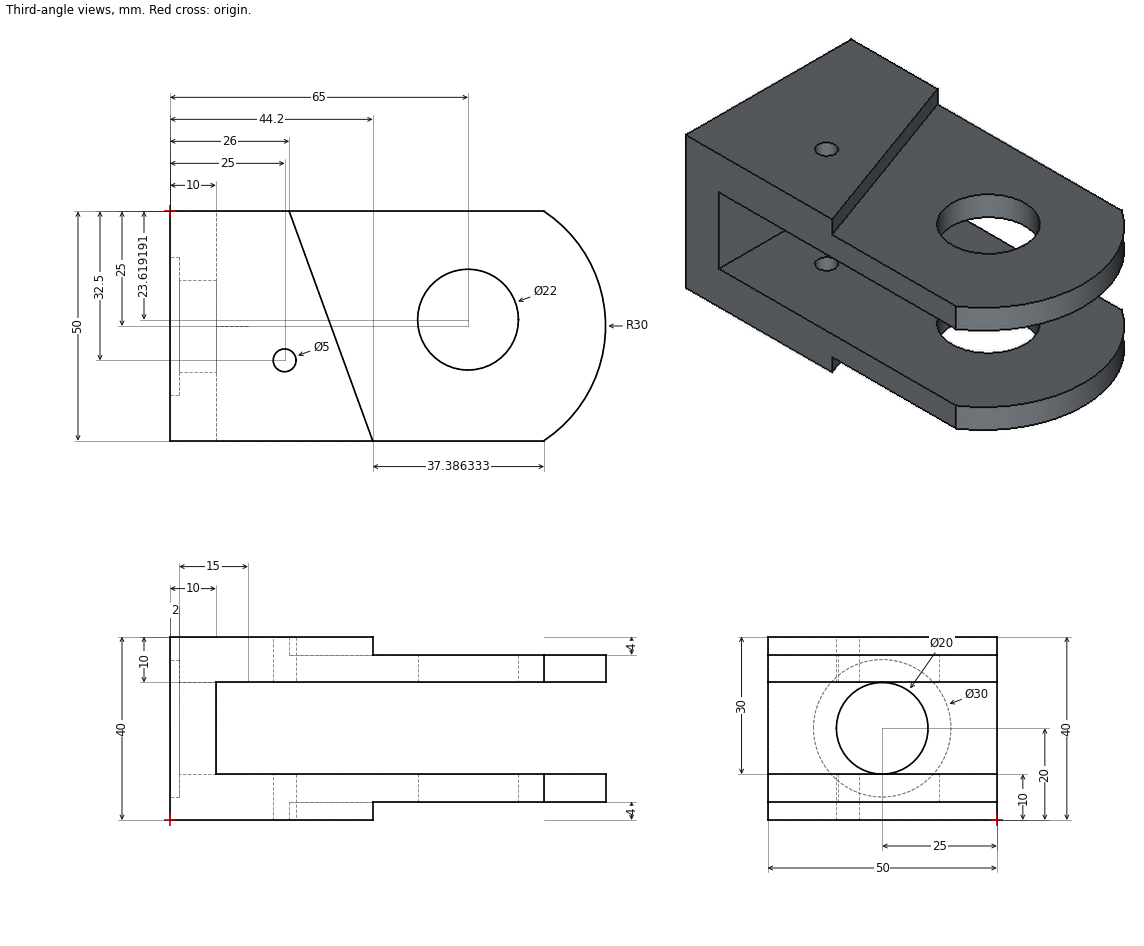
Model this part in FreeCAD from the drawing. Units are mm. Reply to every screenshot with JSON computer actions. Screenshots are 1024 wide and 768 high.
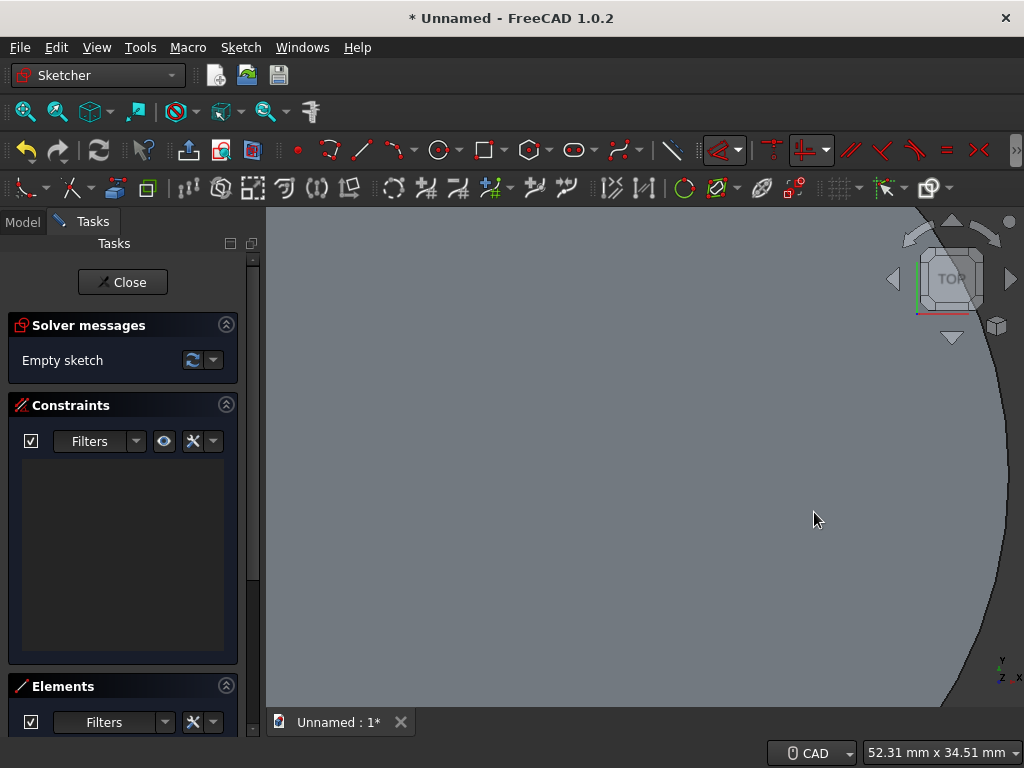
{"action": "left_click", "coordinate": [440, 150]}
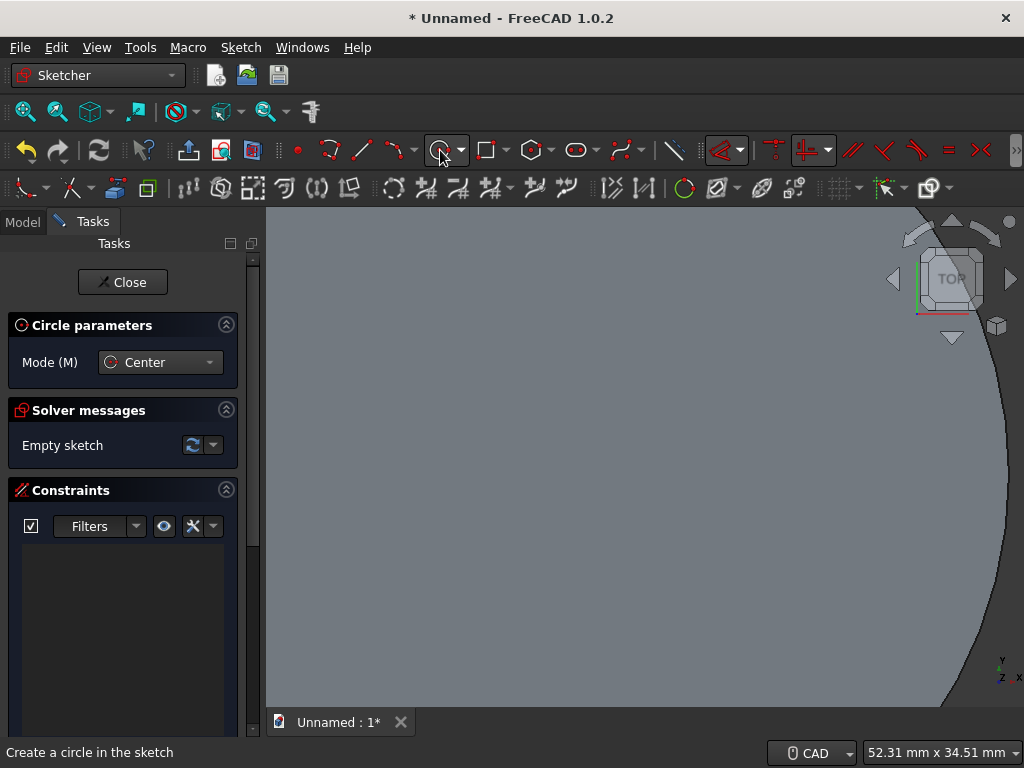
{"action": "left_click", "coordinate": [574, 454]}
{"action": "mouse_move", "coordinate": [687, 342]}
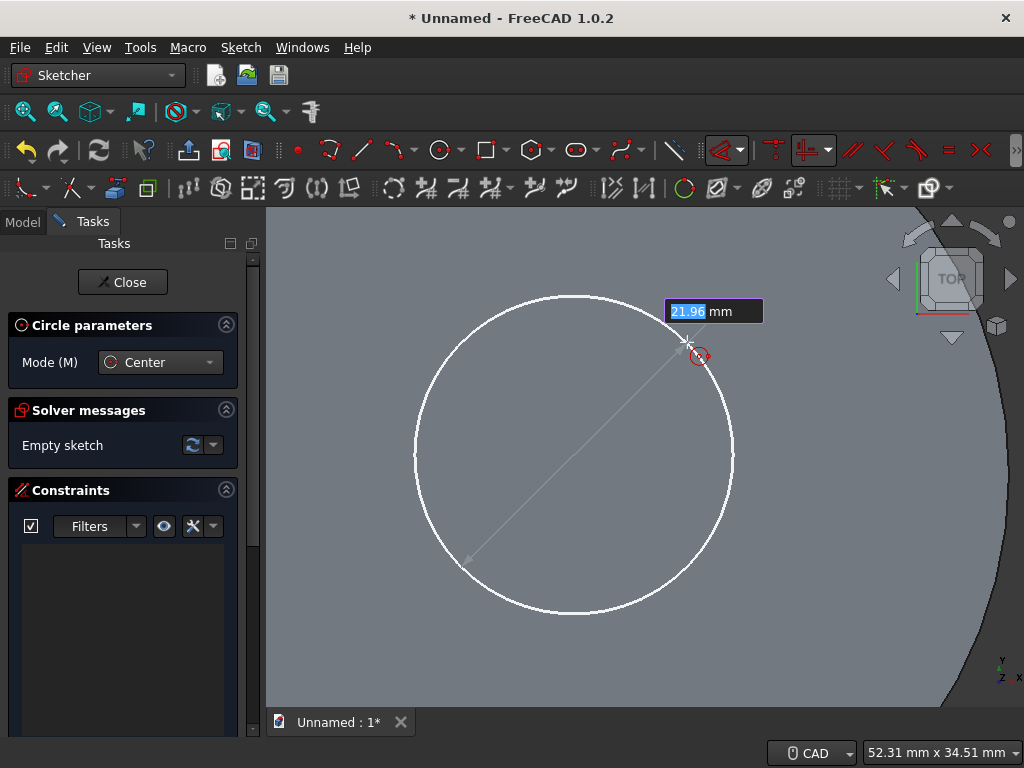
{"action": "type", "text": "22"}
{"action": "key", "text": "Return"}
{"action": "key", "text": "Escape"}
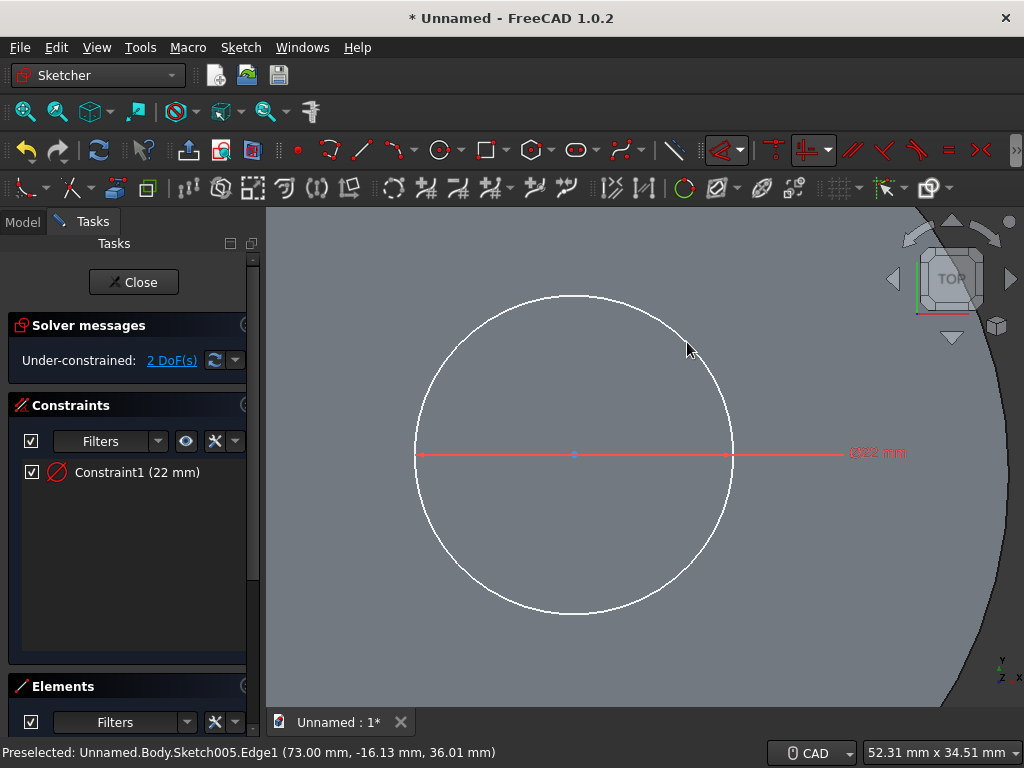
{"action": "left_click", "coordinate": [574, 455]}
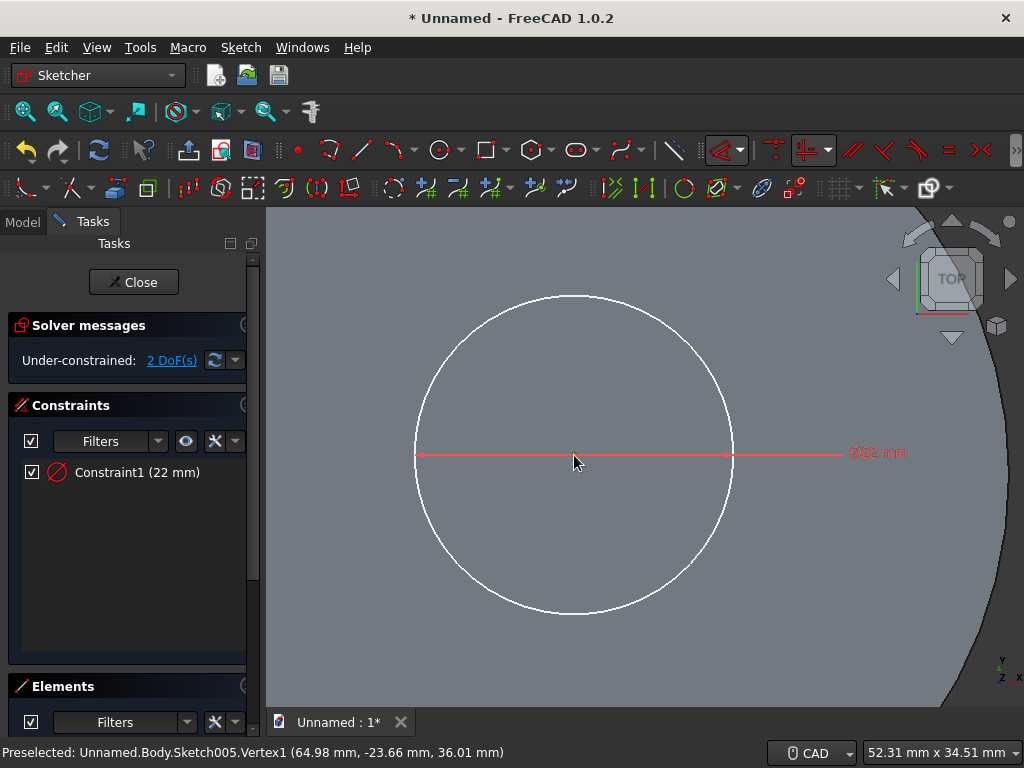
{"action": "key", "text": "l"}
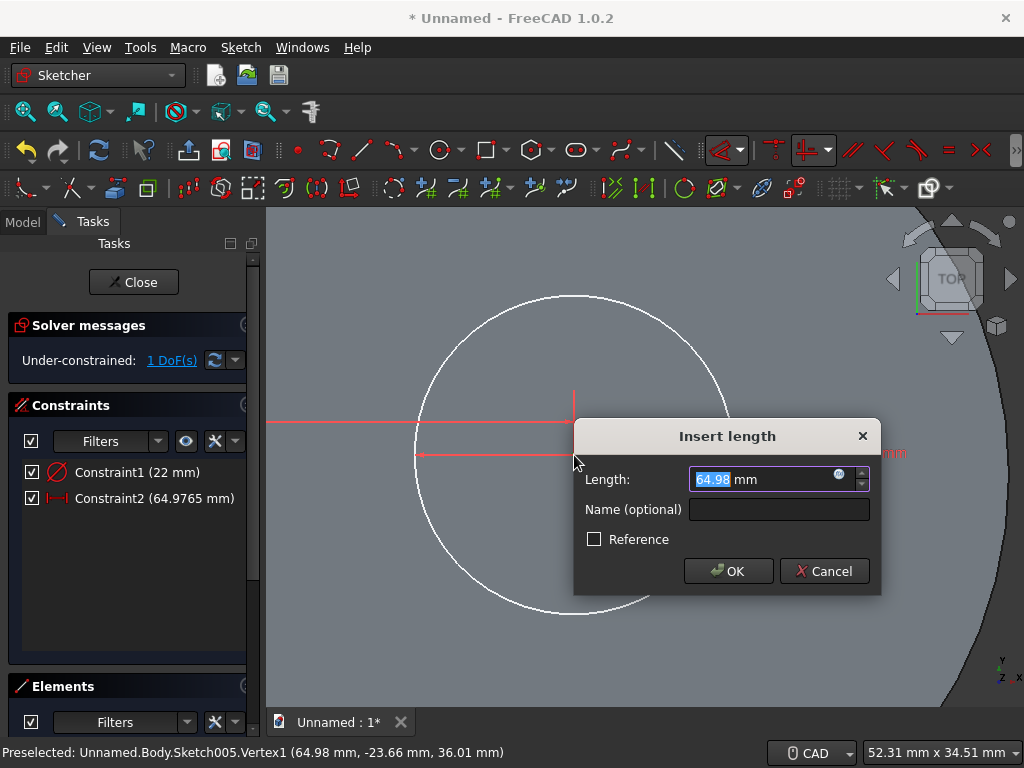
{"action": "type", "text": "65"}
{"action": "key", "text": "Return"}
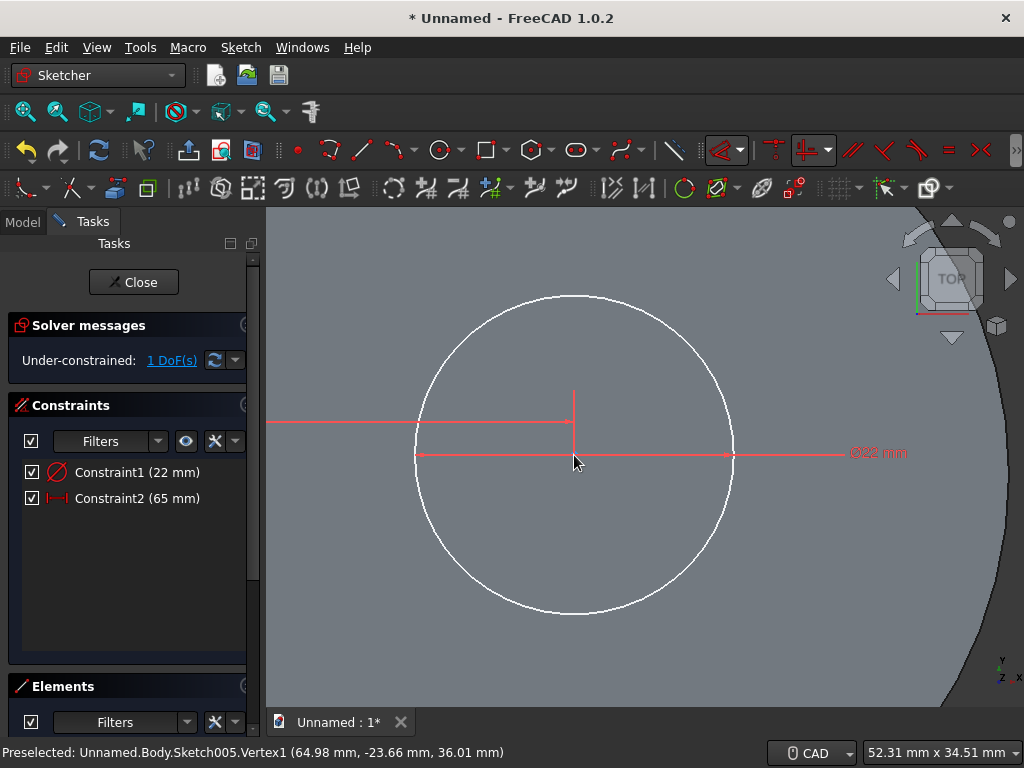
{"action": "left_click", "coordinate": [574, 455]}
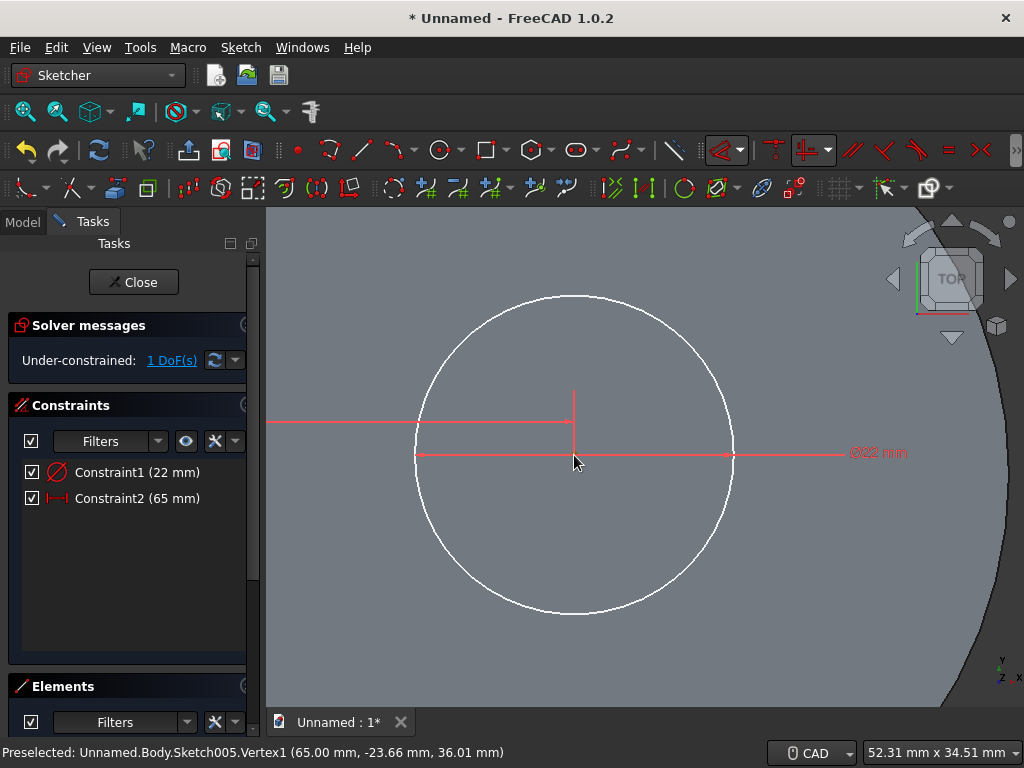
{"action": "key", "text": "i"}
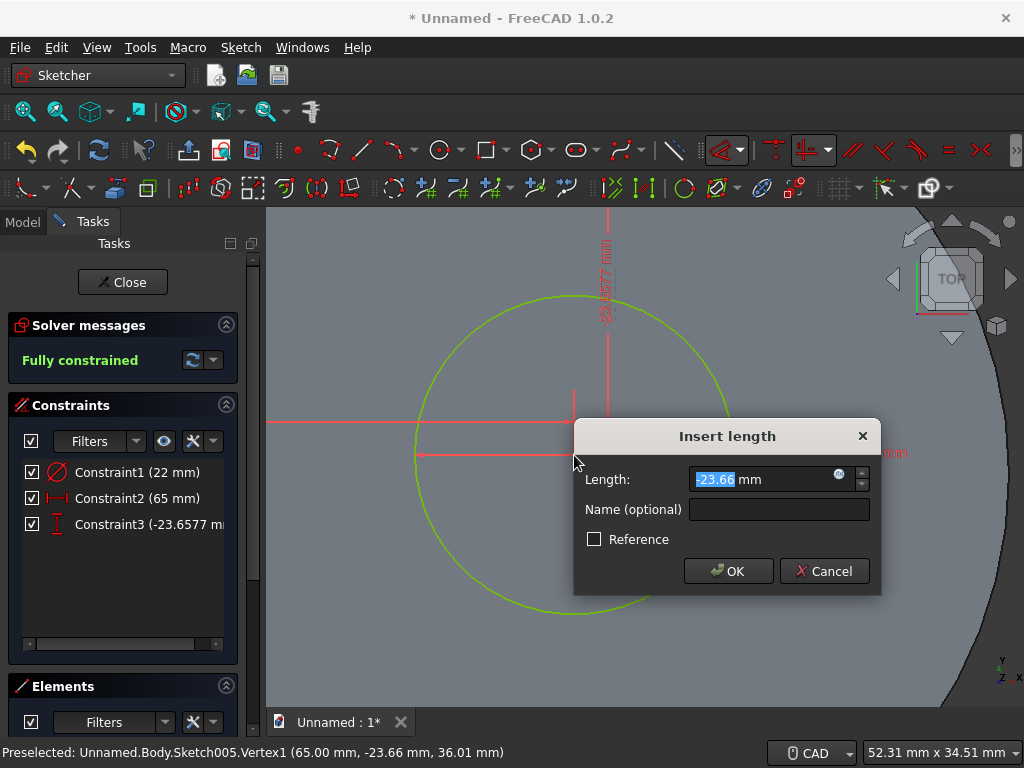
{"action": "type", "text": "-23.619191"}
{"action": "key", "text": "Return"}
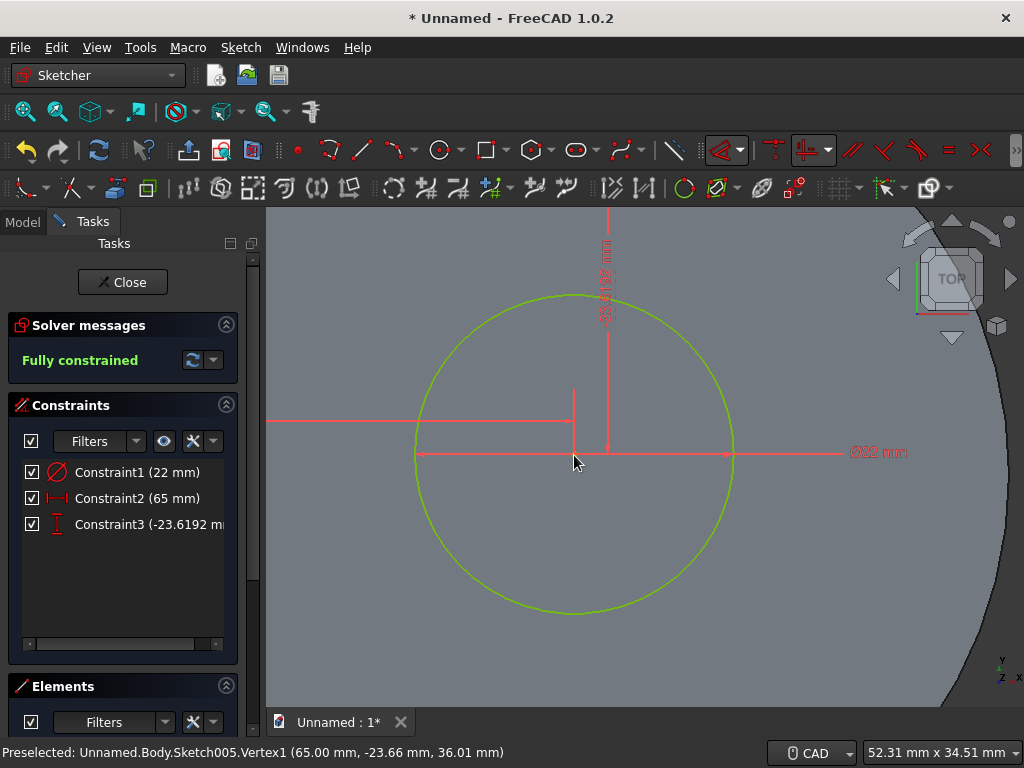
{"action": "left_click", "coordinate": [123, 282]}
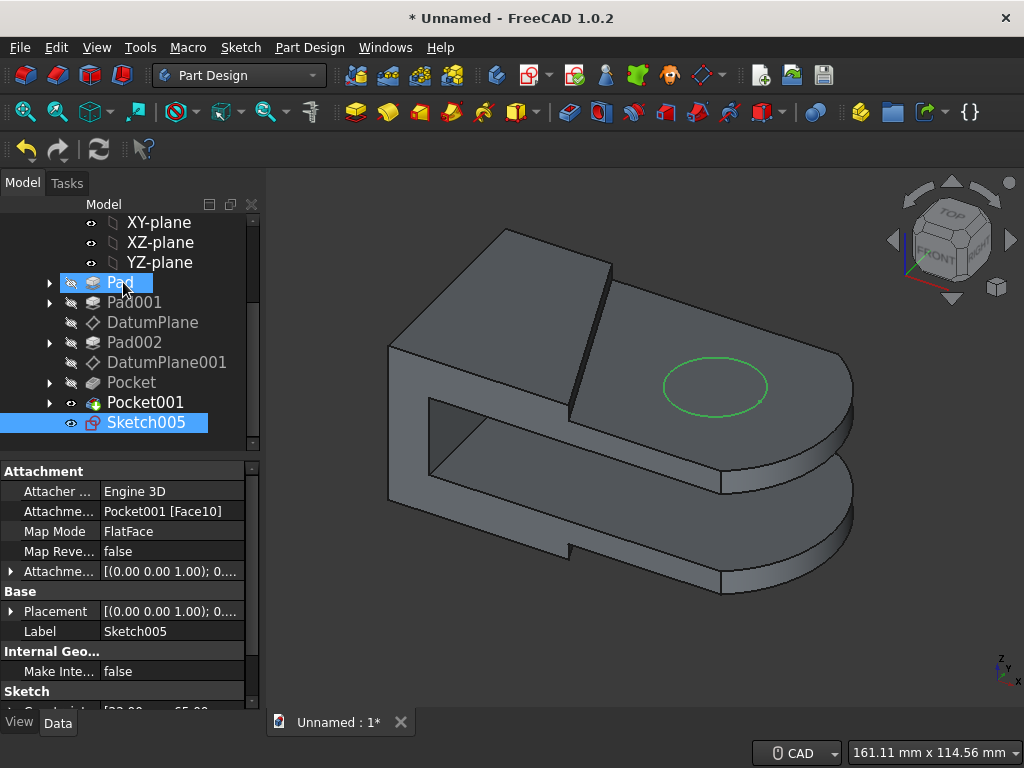
{"action": "left_click", "coordinate": [570, 112]}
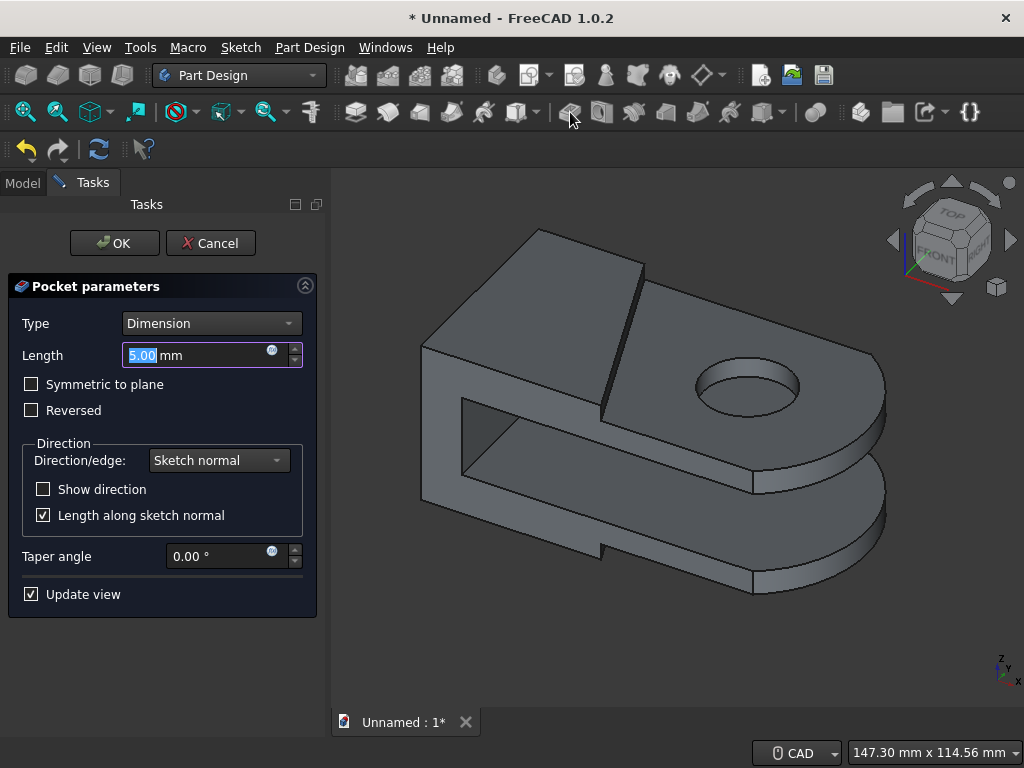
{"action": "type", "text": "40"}
{"action": "key", "text": "Tab"}